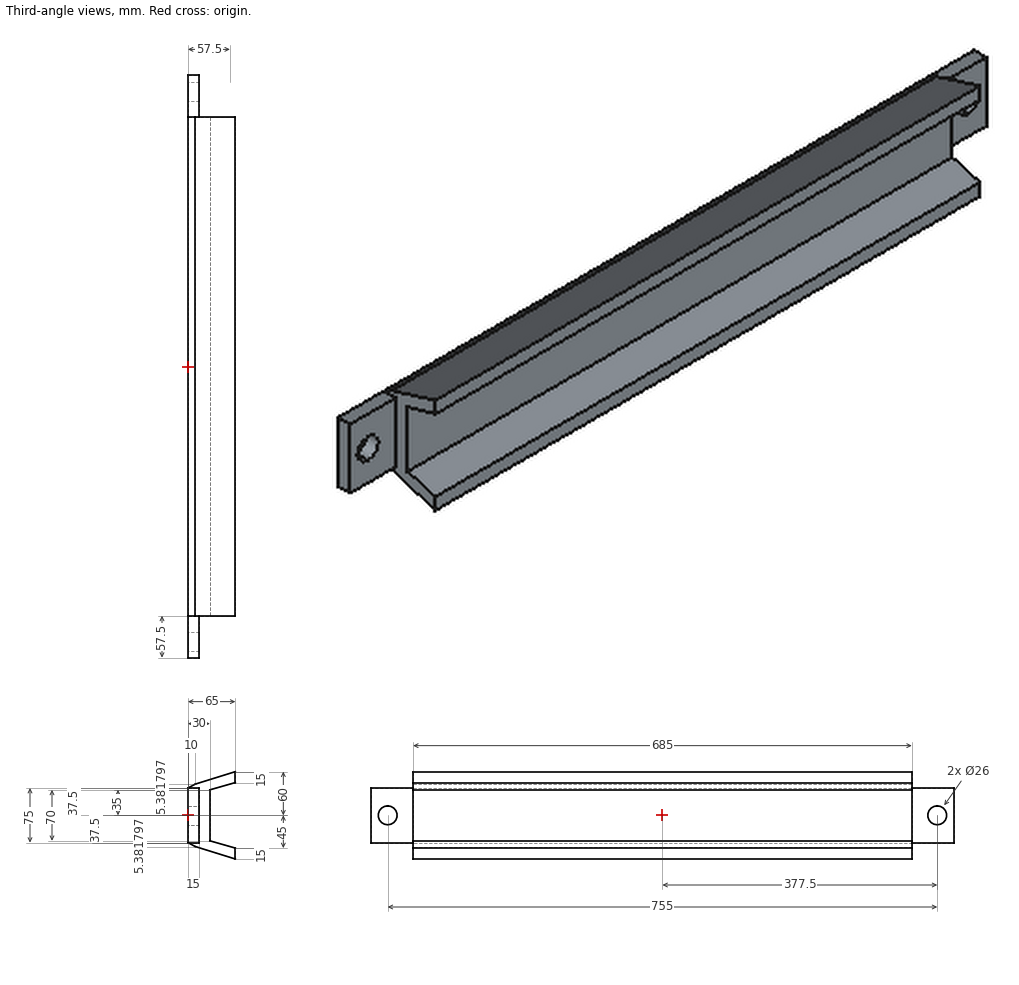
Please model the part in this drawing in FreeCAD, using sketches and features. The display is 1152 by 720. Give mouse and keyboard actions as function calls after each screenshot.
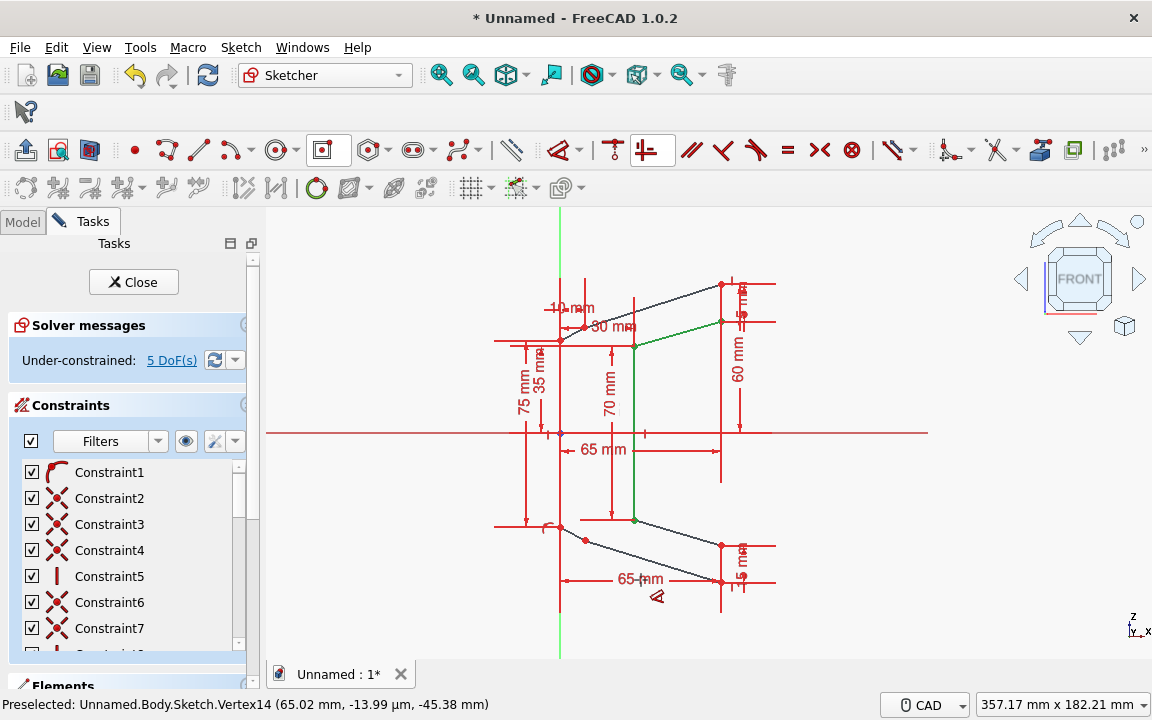
click(721, 546)
click(755, 490)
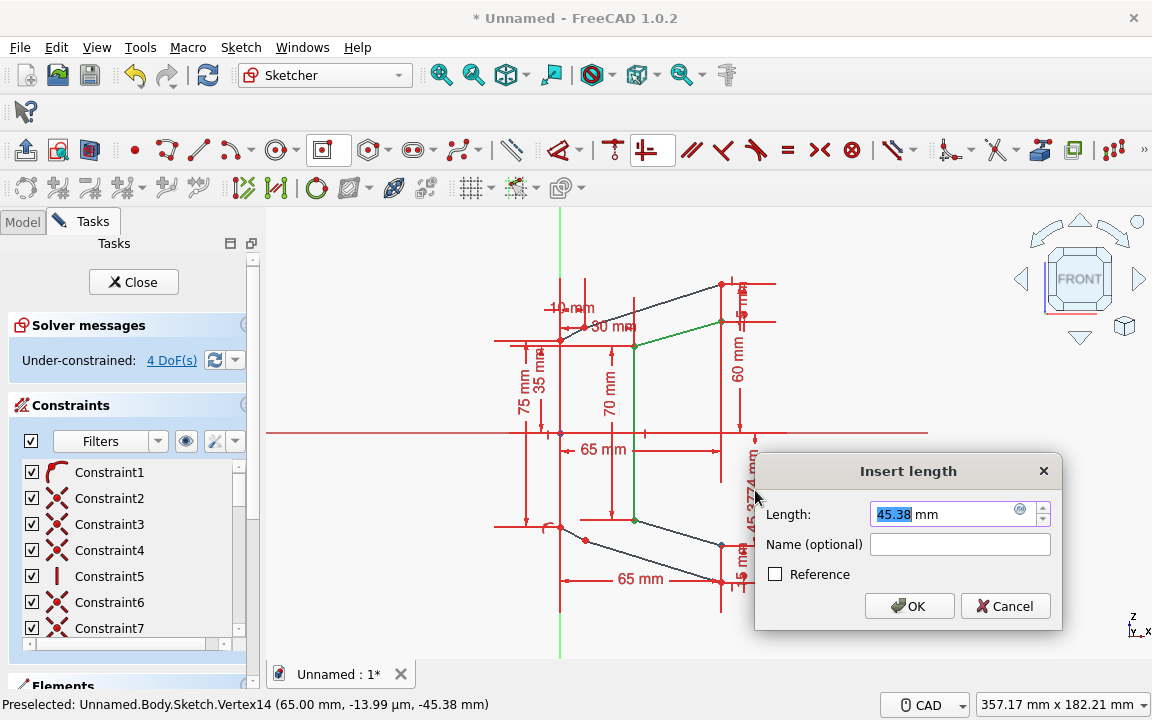
text(45)
key(Return)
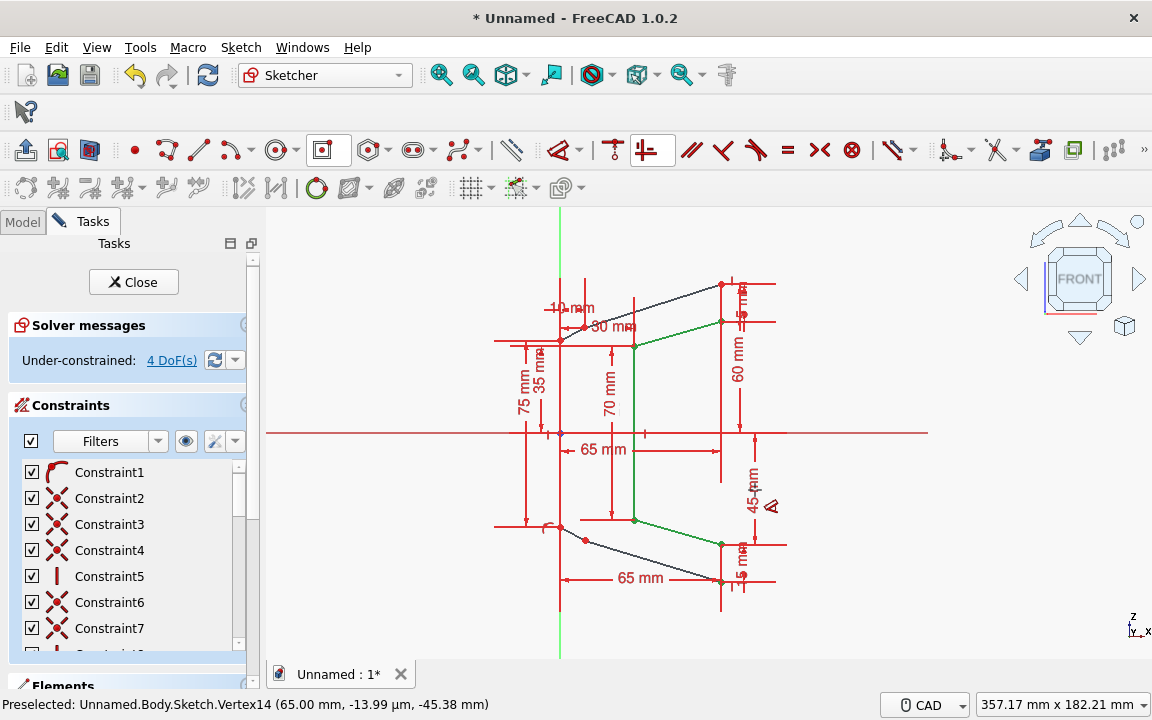
scroll(585, 541, up, 3)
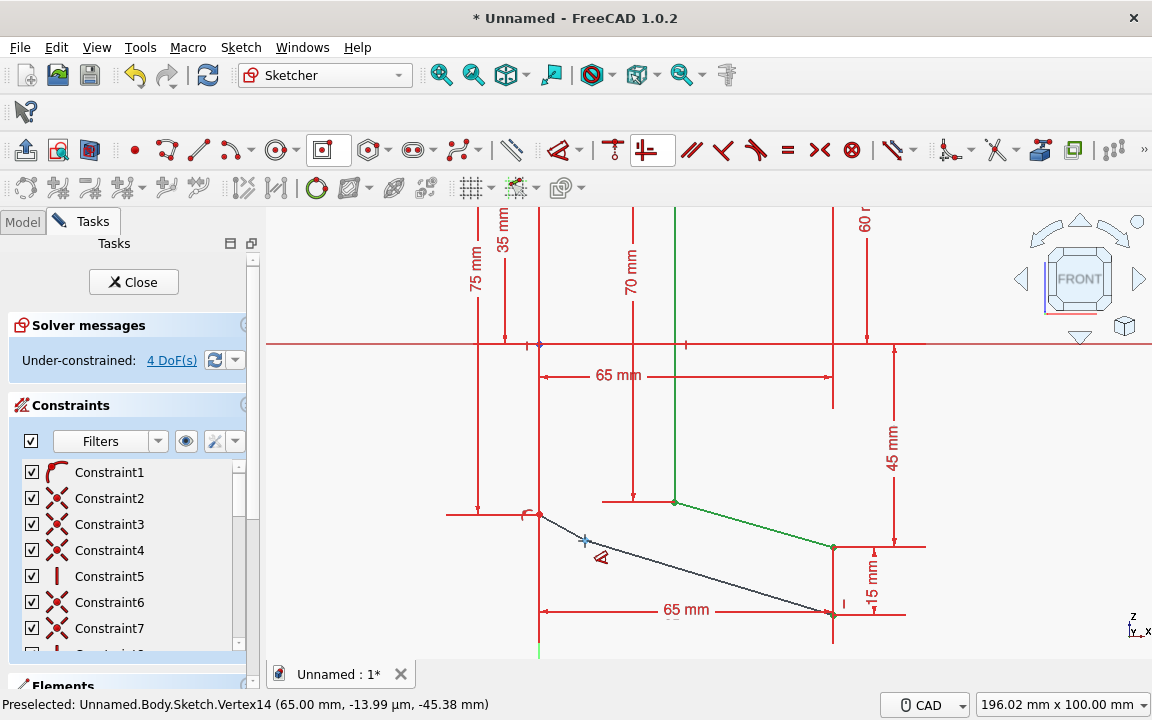
click(585, 540)
click(562, 574)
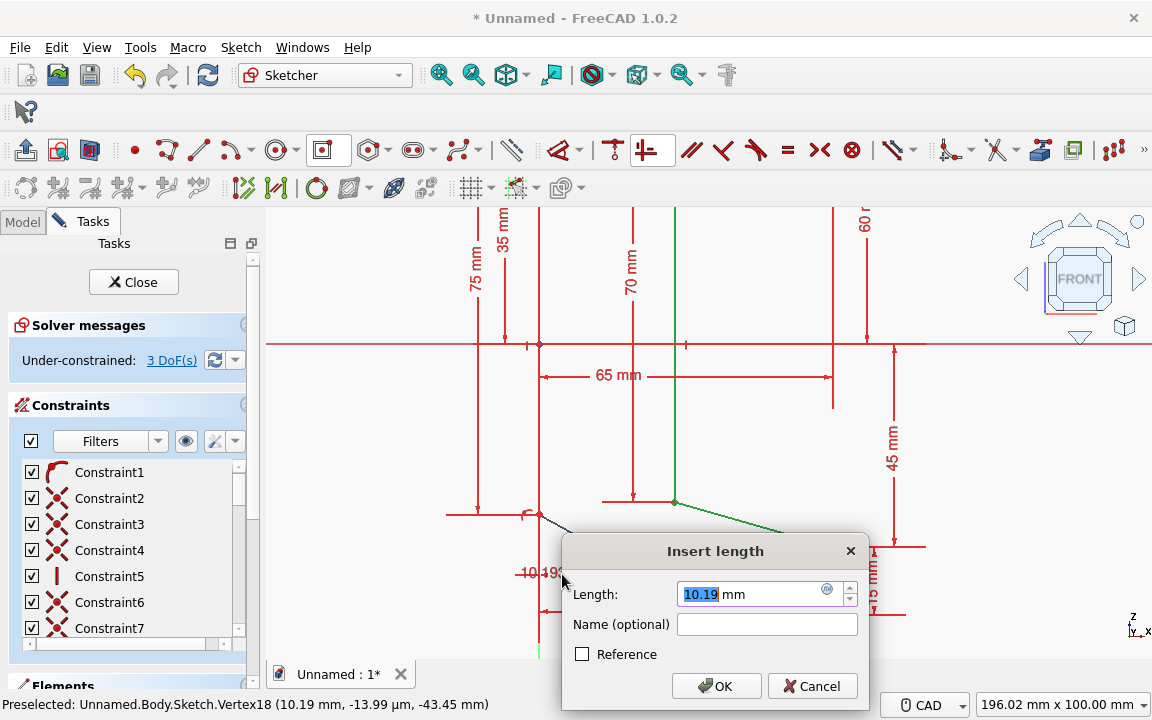
text(10)
key(Return)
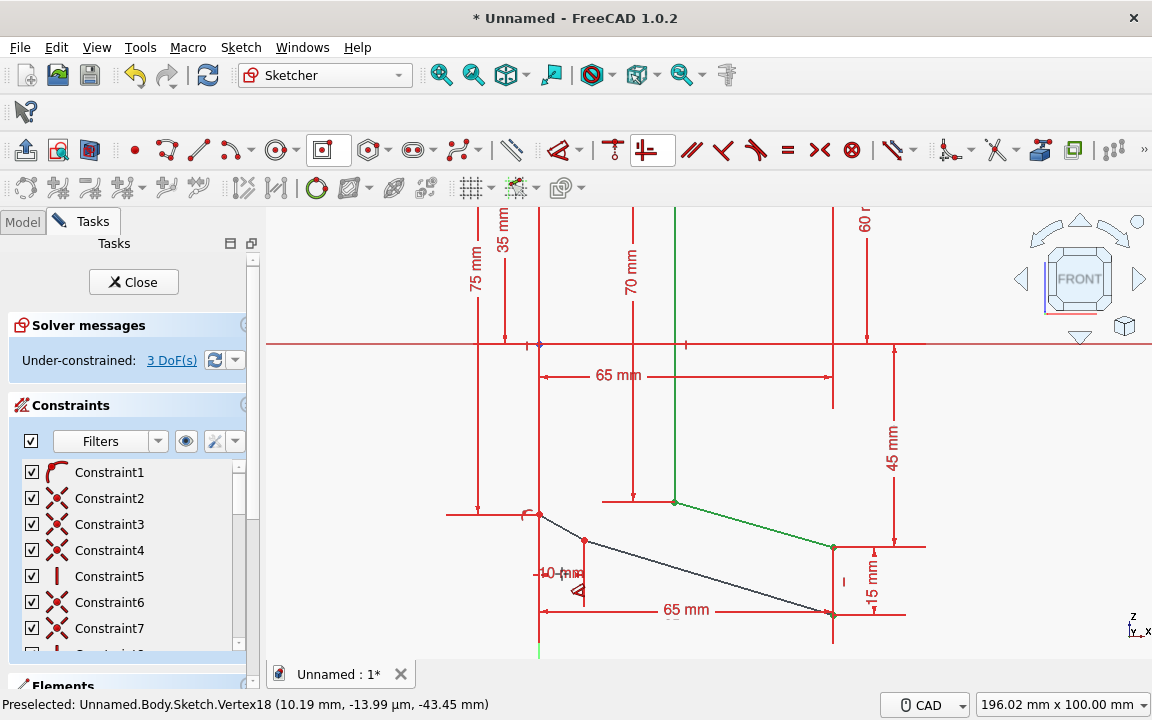
click(539, 515)
click(505, 429)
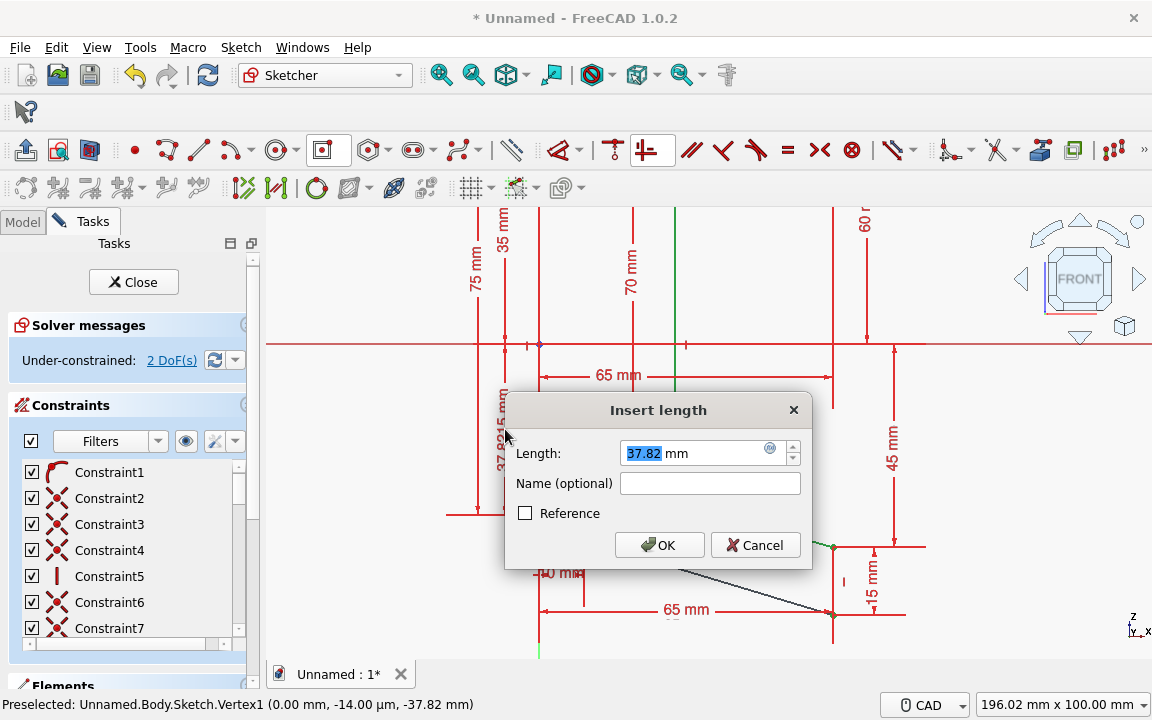
text(37.5)
key(Return)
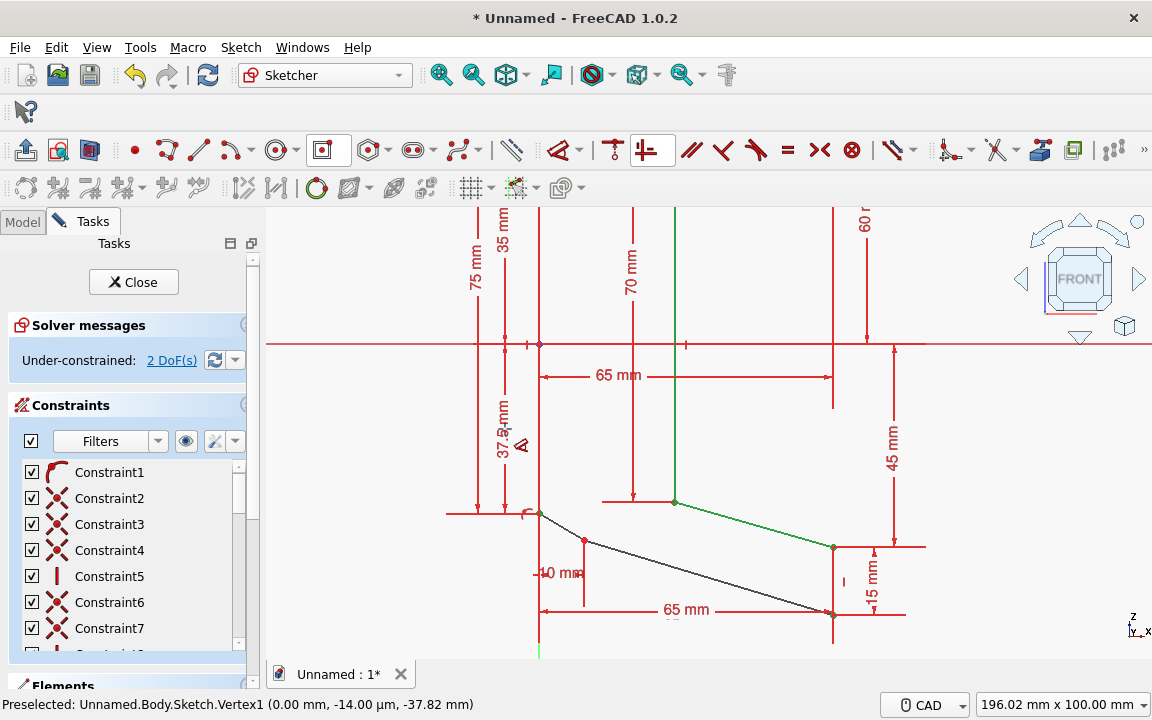
scroll(585, 541, down, 3)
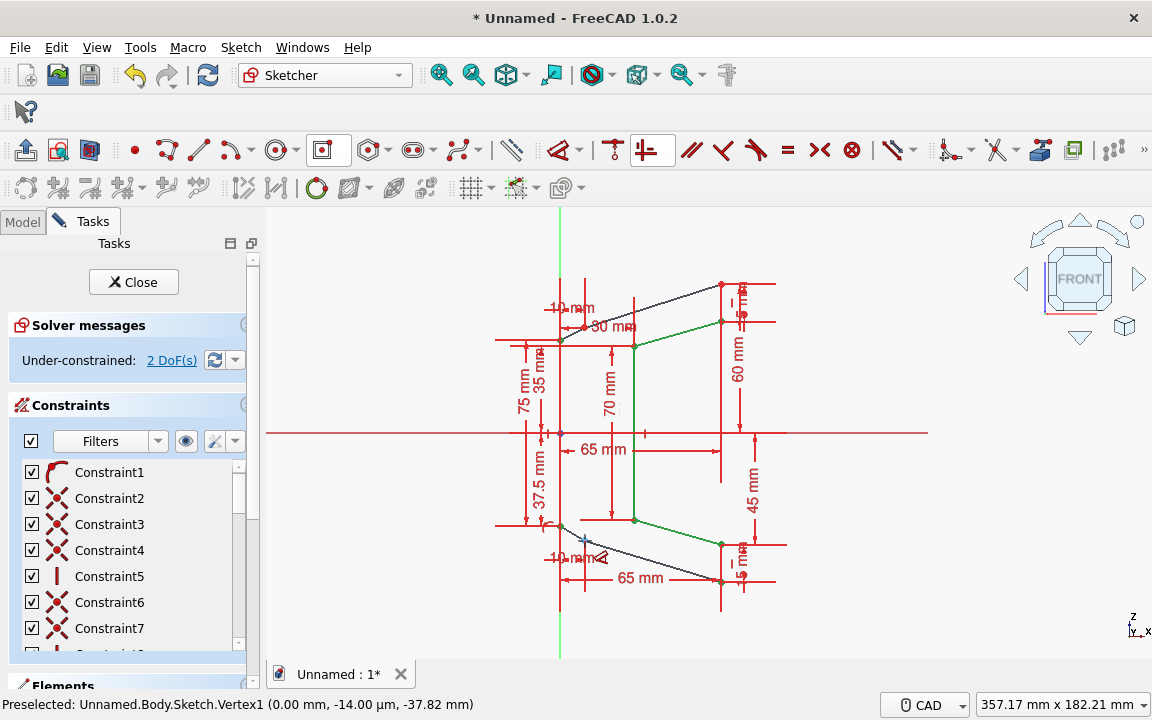
scroll(567, 337, up, 6)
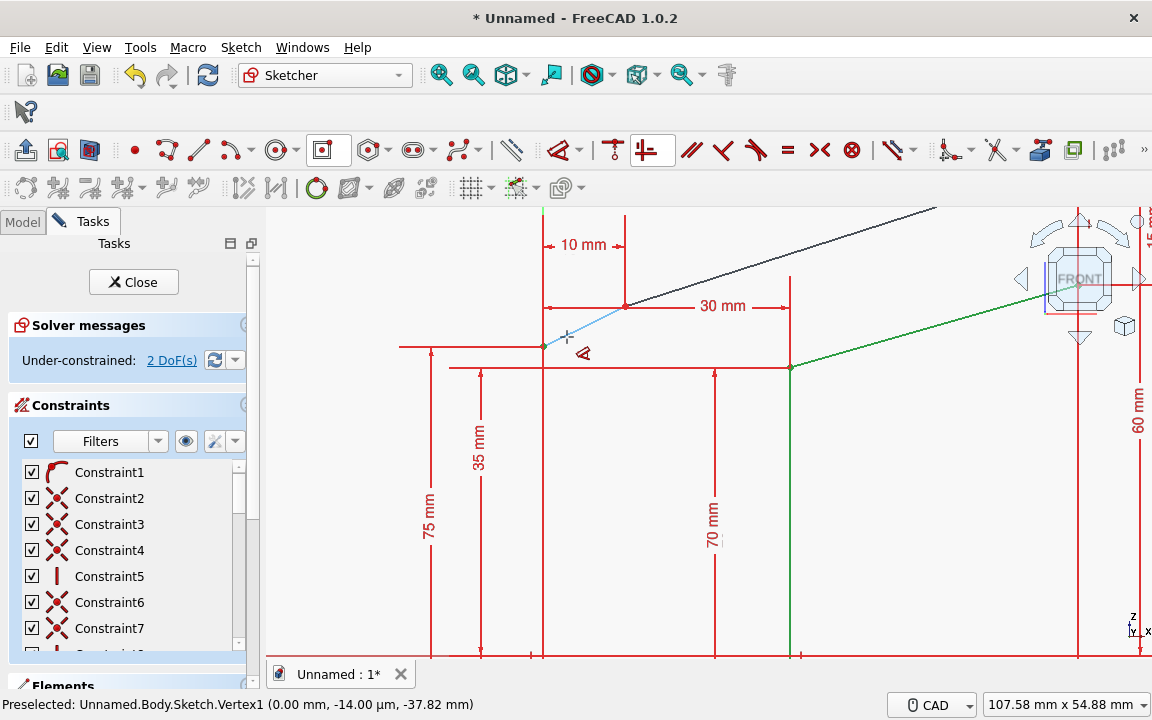
click(568, 335)
click(509, 327)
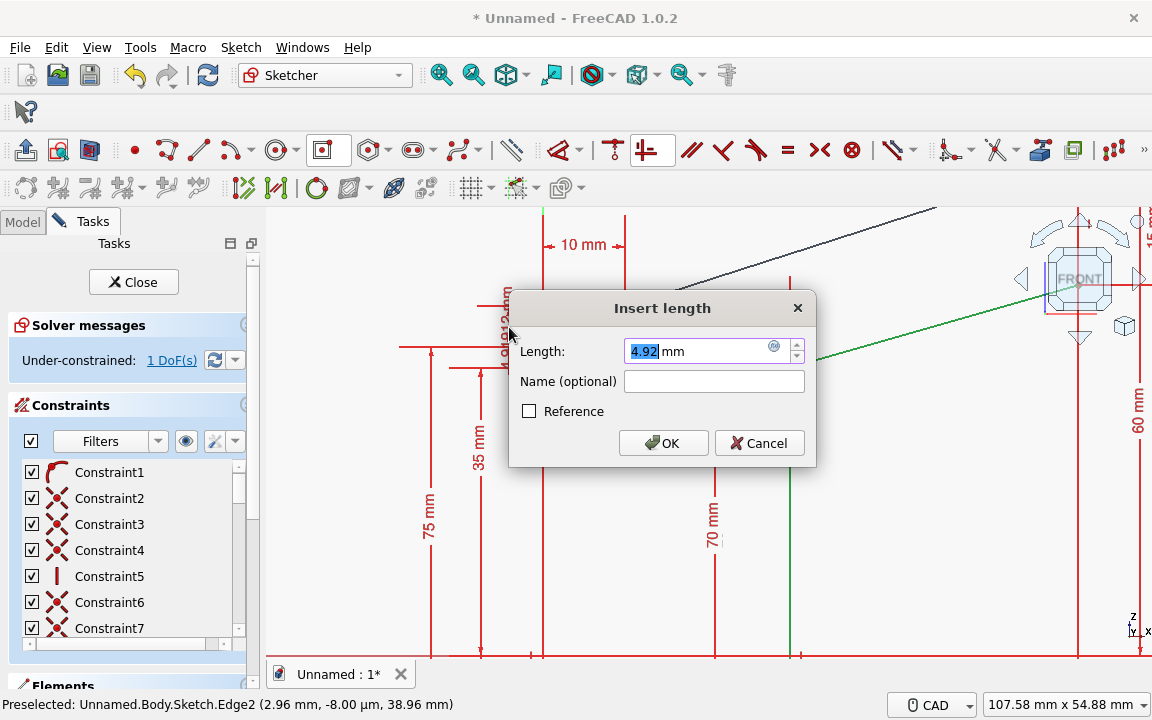
text(5.381797)
key(Return)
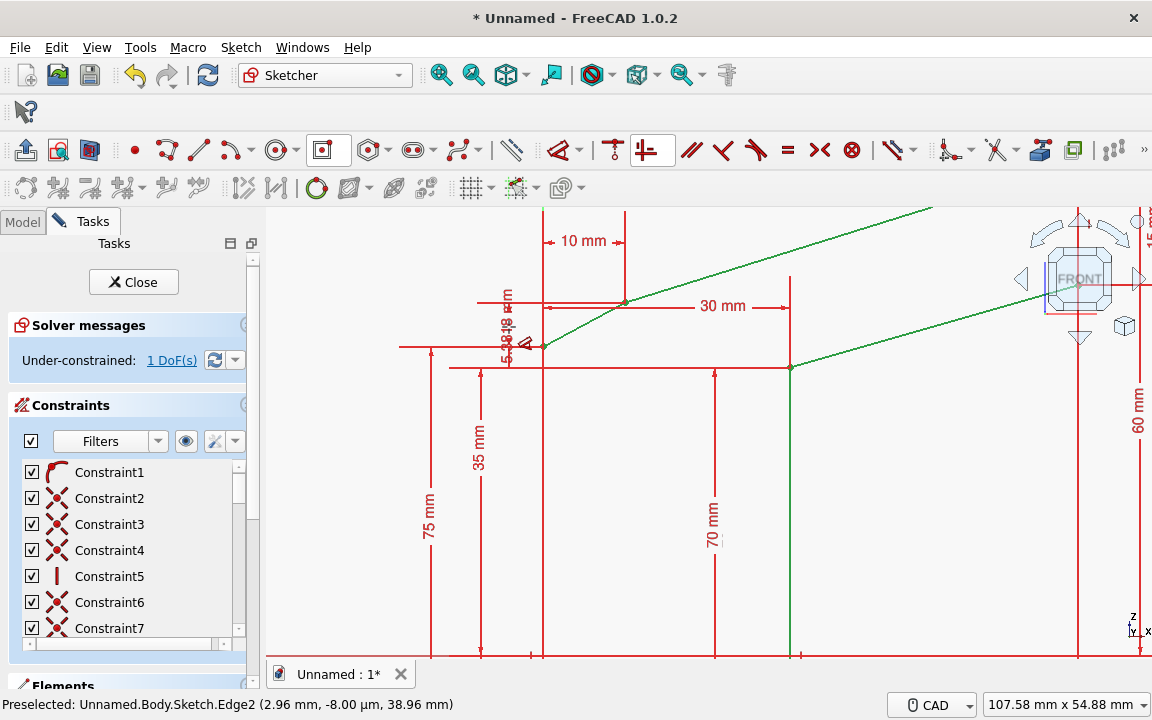
scroll(567, 337, down, 6)